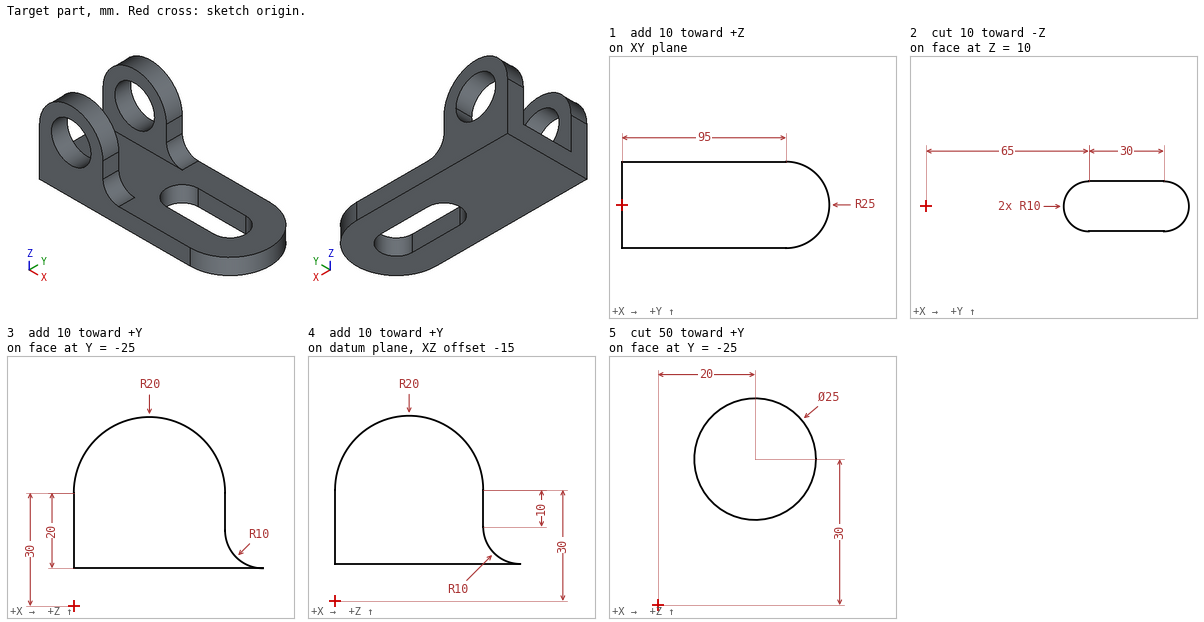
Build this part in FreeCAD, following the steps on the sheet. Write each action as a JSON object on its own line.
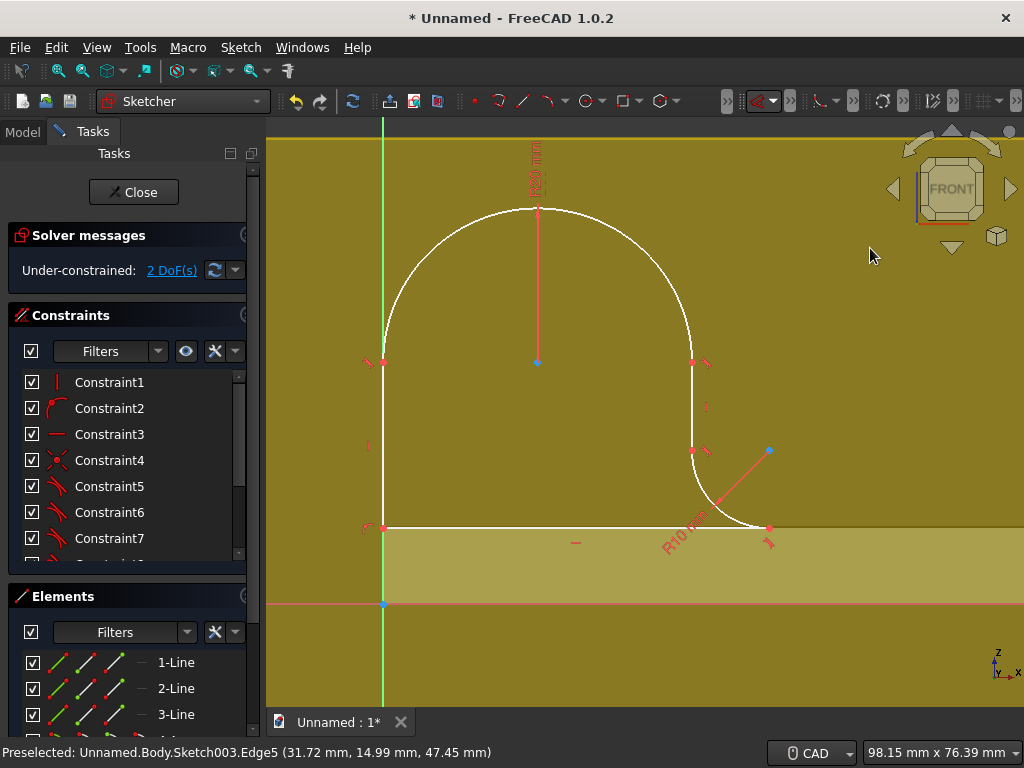
{"action": "left_click", "coordinate": [692, 389]}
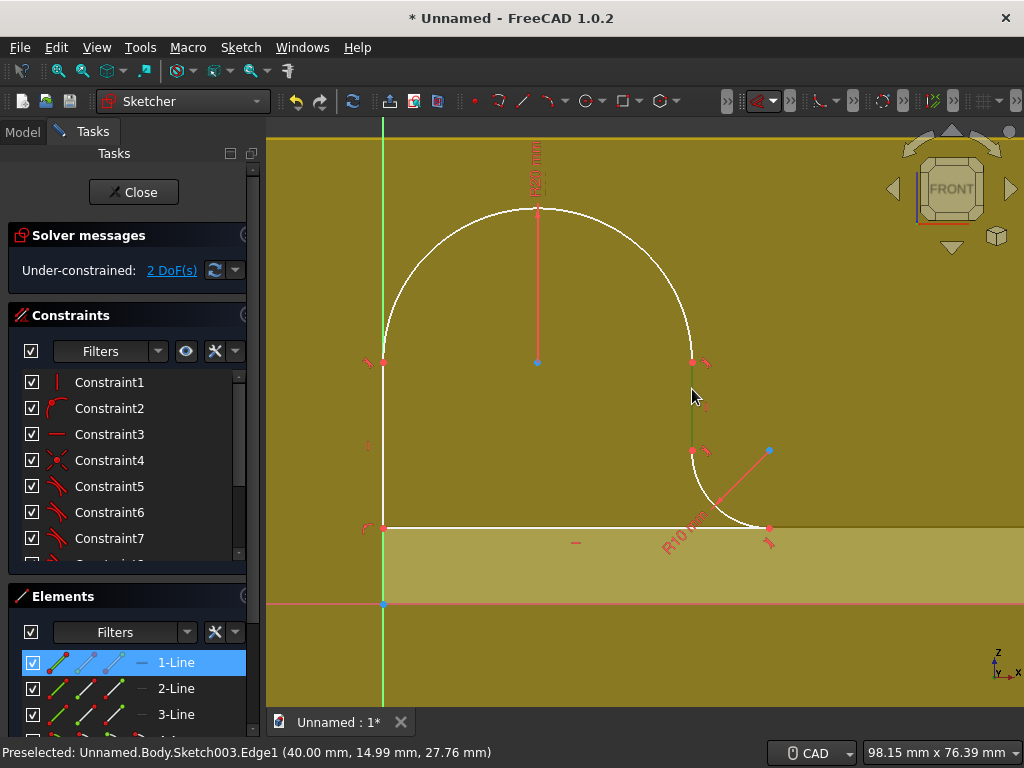
{"action": "left_click", "coordinate": [776, 102]}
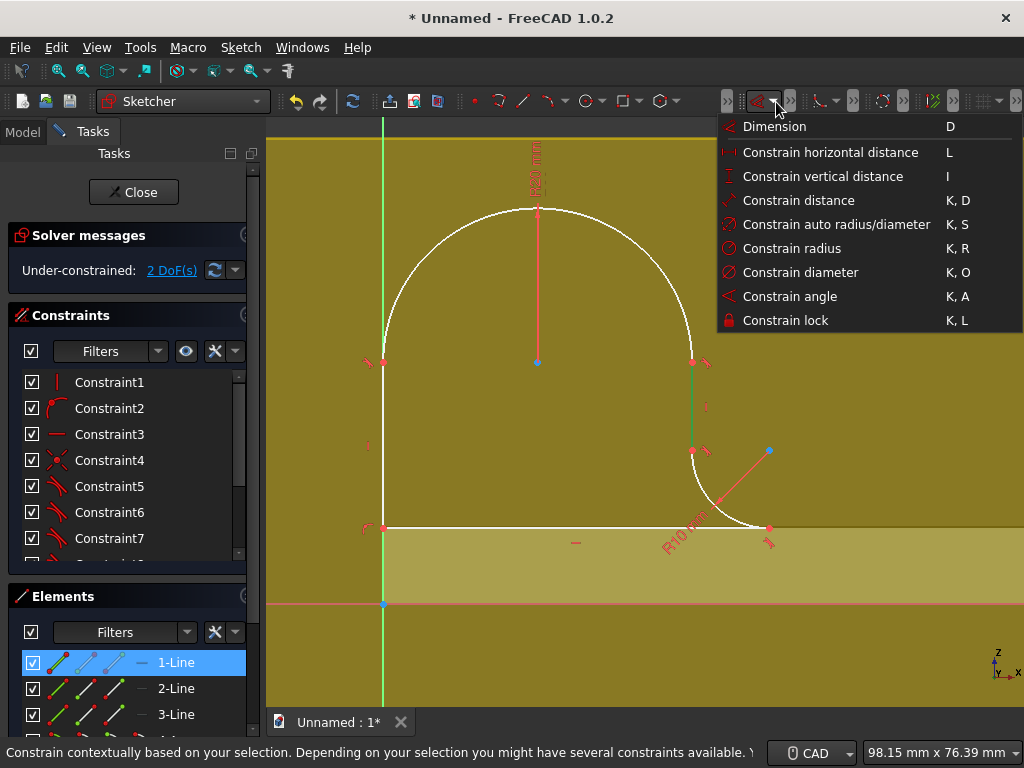
{"action": "left_click", "coordinate": [870, 176]}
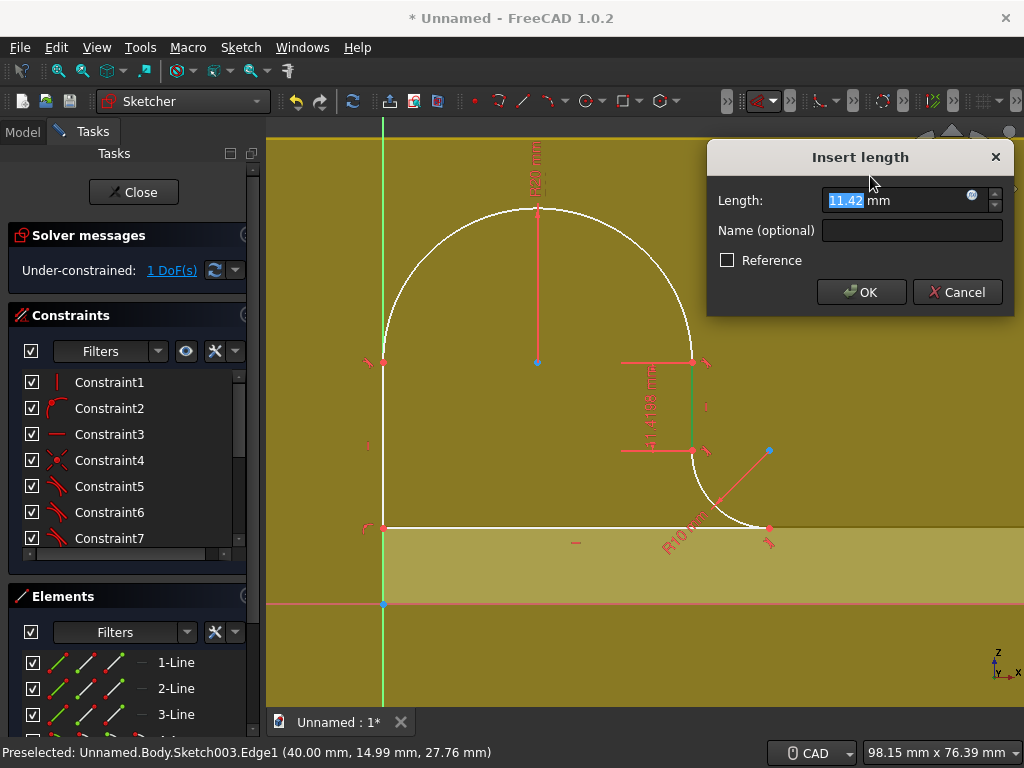
{"action": "type", "text": "10"}
{"action": "key", "text": "Return"}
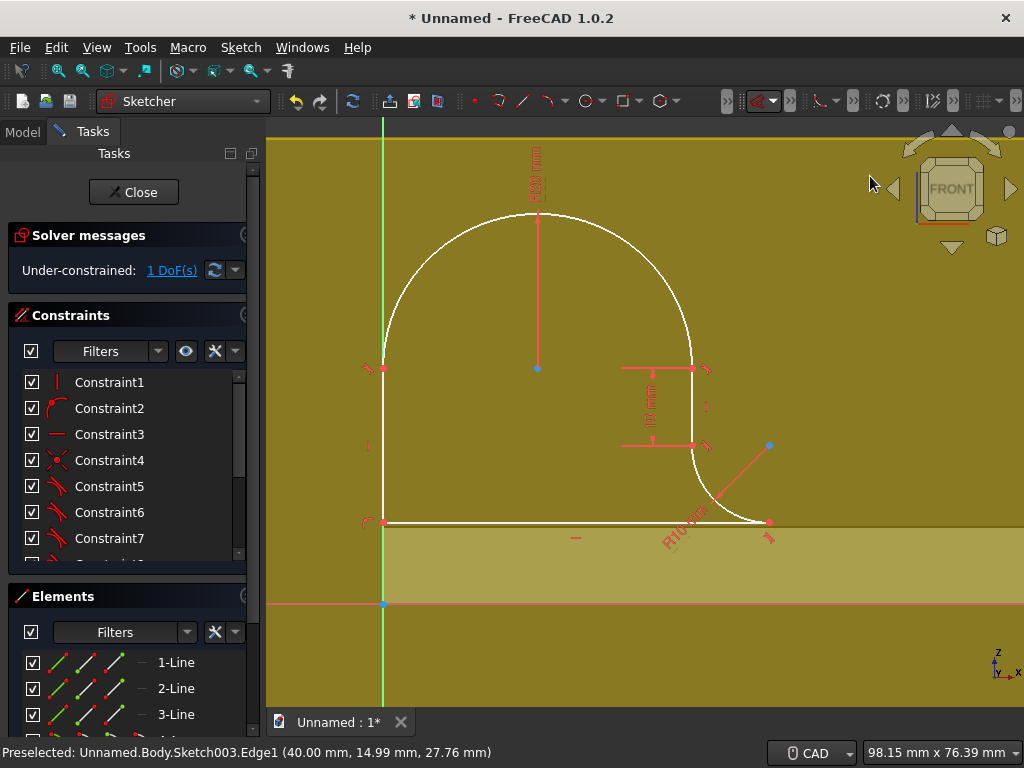
{"action": "left_click", "coordinate": [692, 368]}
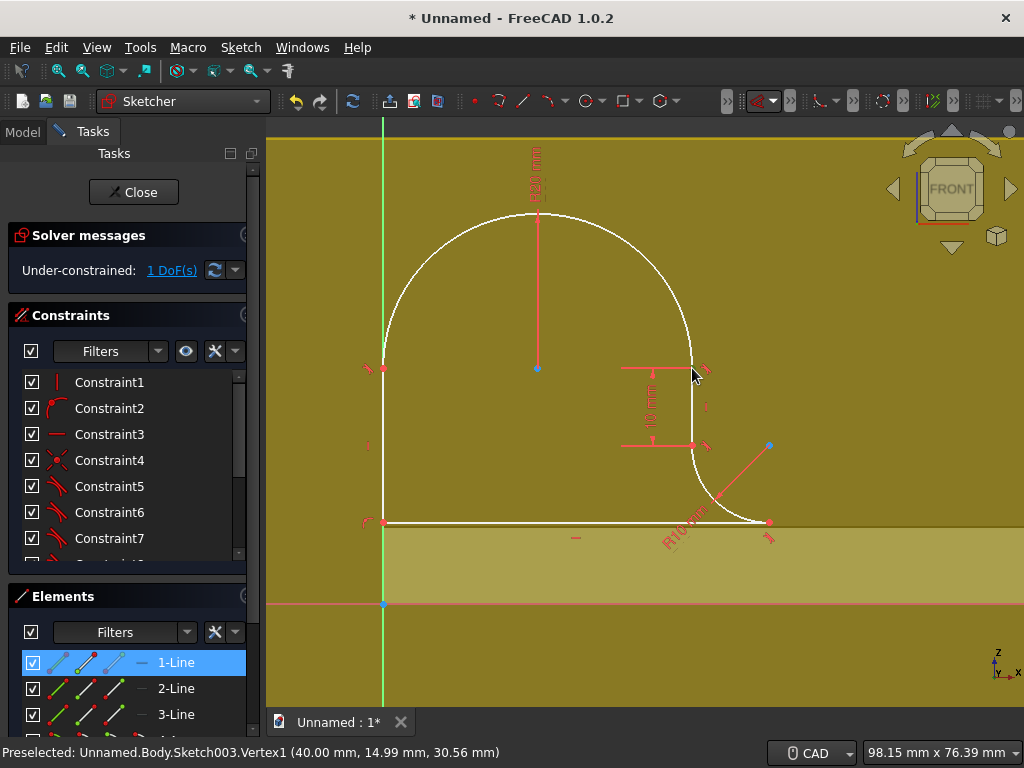
{"action": "left_click", "coordinate": [776, 102]}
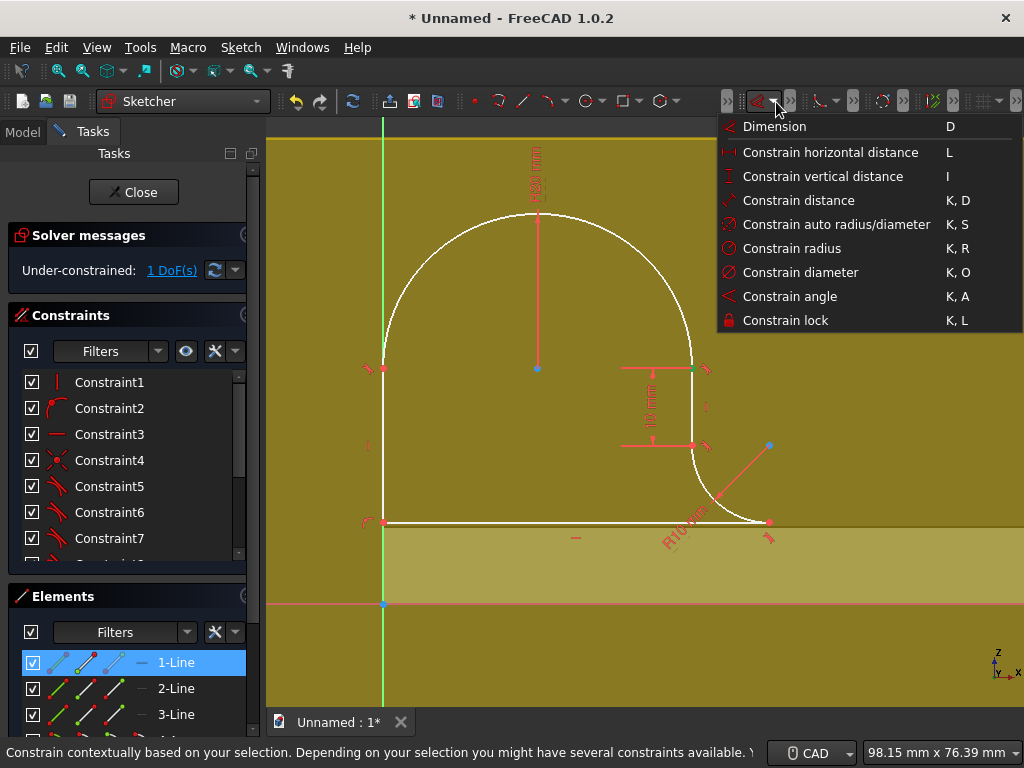
{"action": "left_click", "coordinate": [870, 176]}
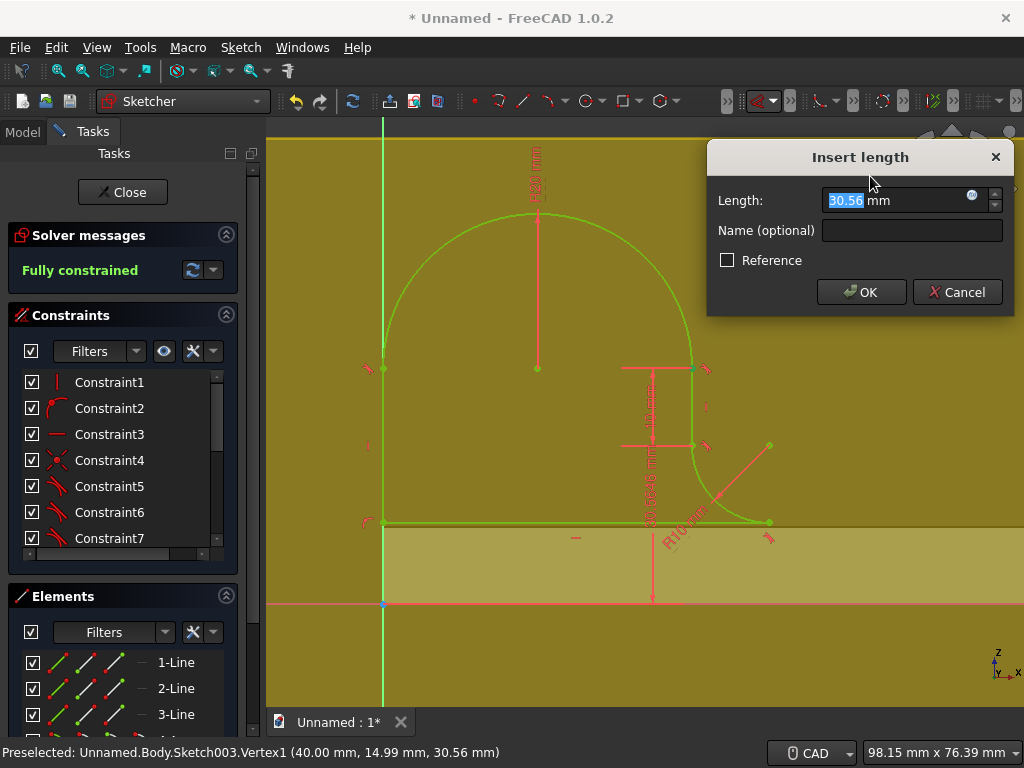
{"action": "type", "text": "30"}
{"action": "key", "text": "Return"}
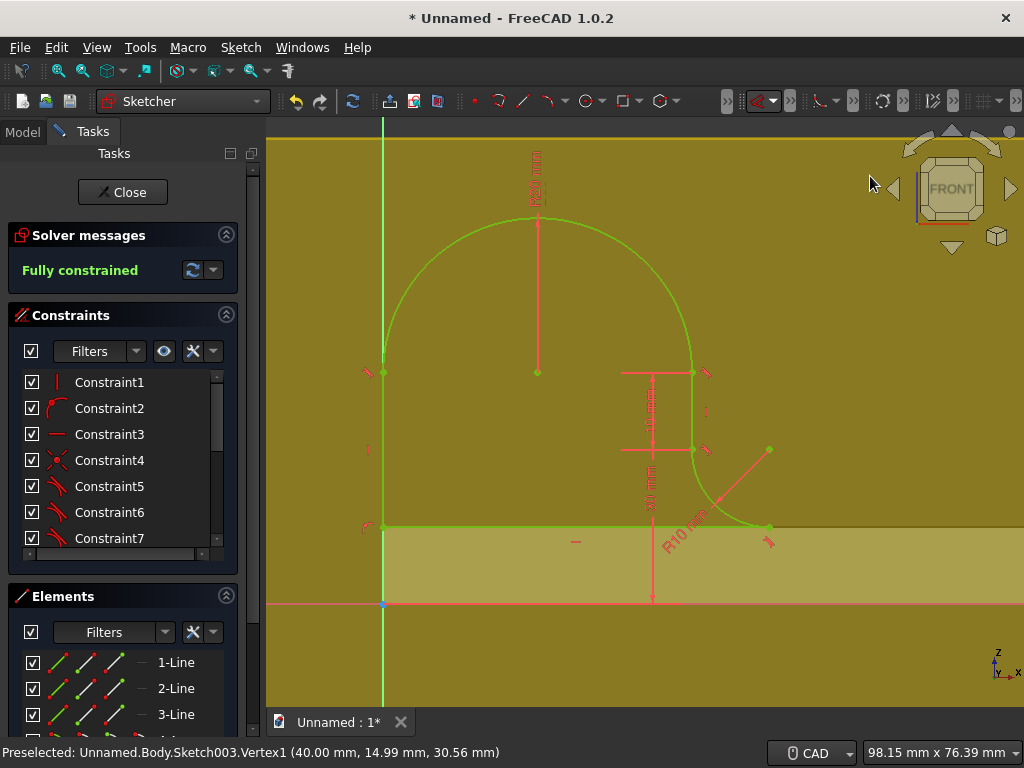
{"action": "left_click", "coordinate": [123, 192]}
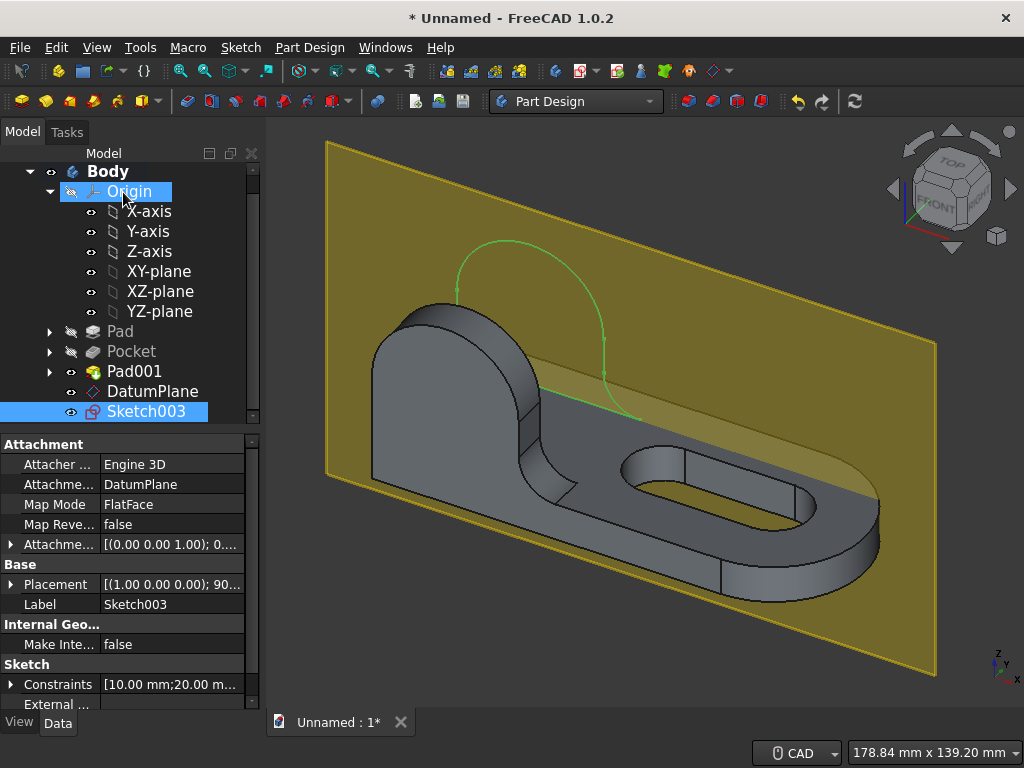
{"action": "left_click", "coordinate": [22, 102]}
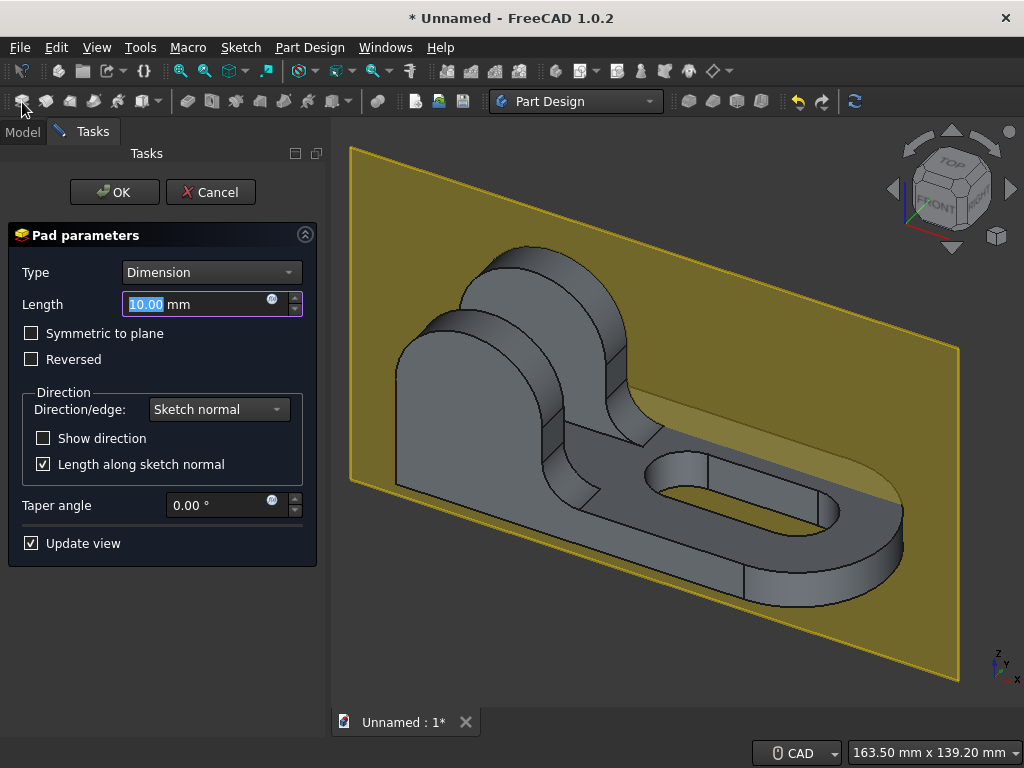
{"action": "type", "text": "10"}
{"action": "key", "text": "Tab"}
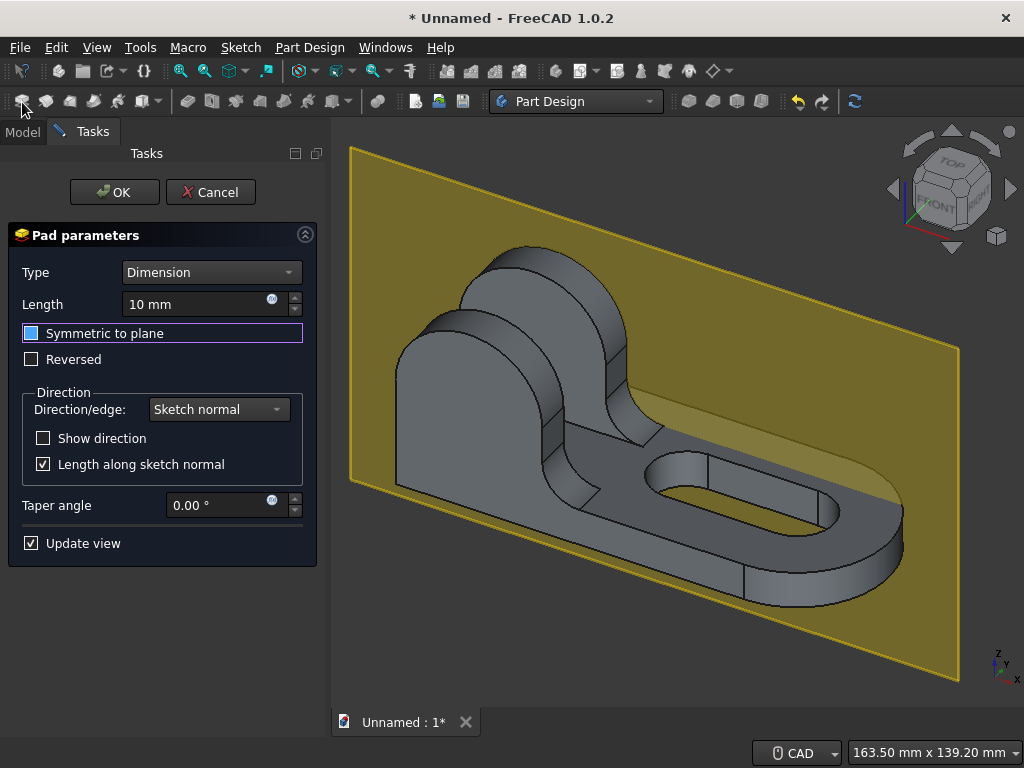
{"action": "left_click", "coordinate": [30, 359]}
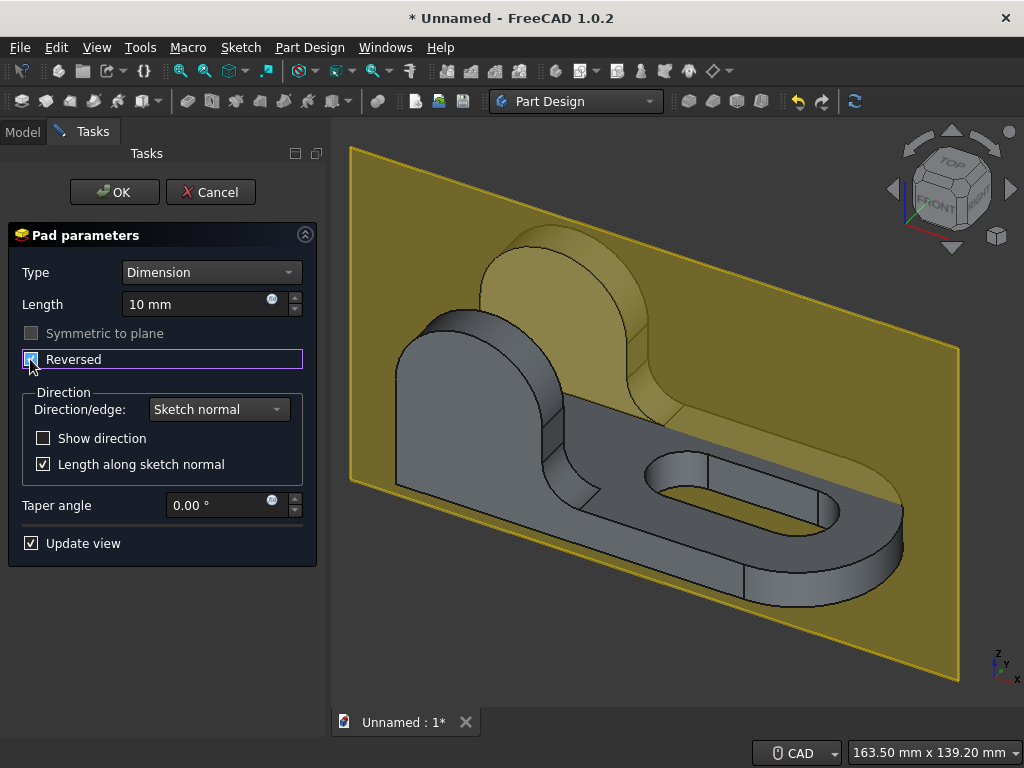
{"action": "left_click", "coordinate": [115, 192]}